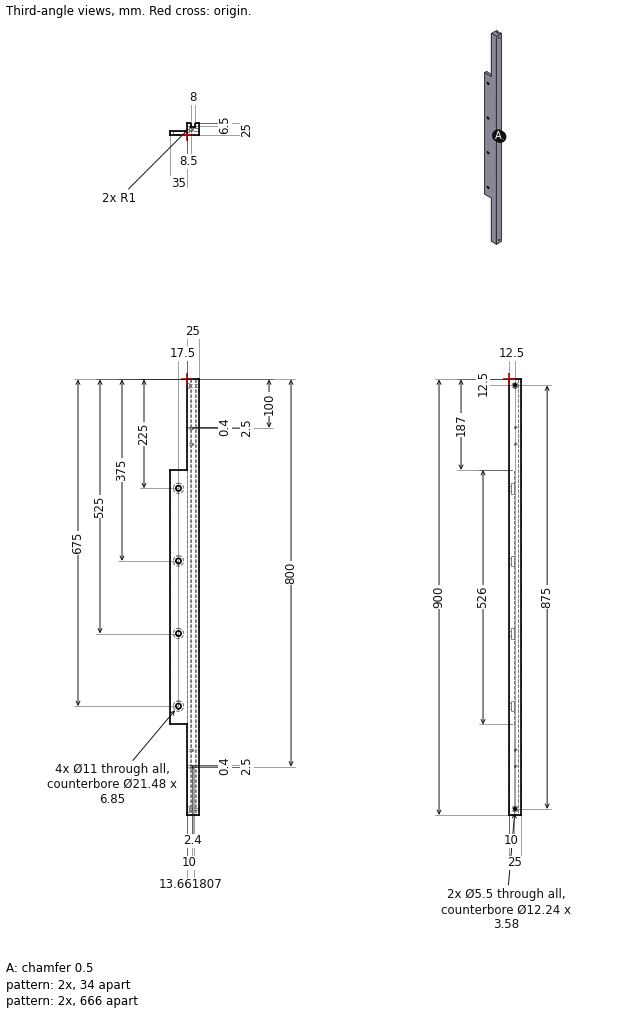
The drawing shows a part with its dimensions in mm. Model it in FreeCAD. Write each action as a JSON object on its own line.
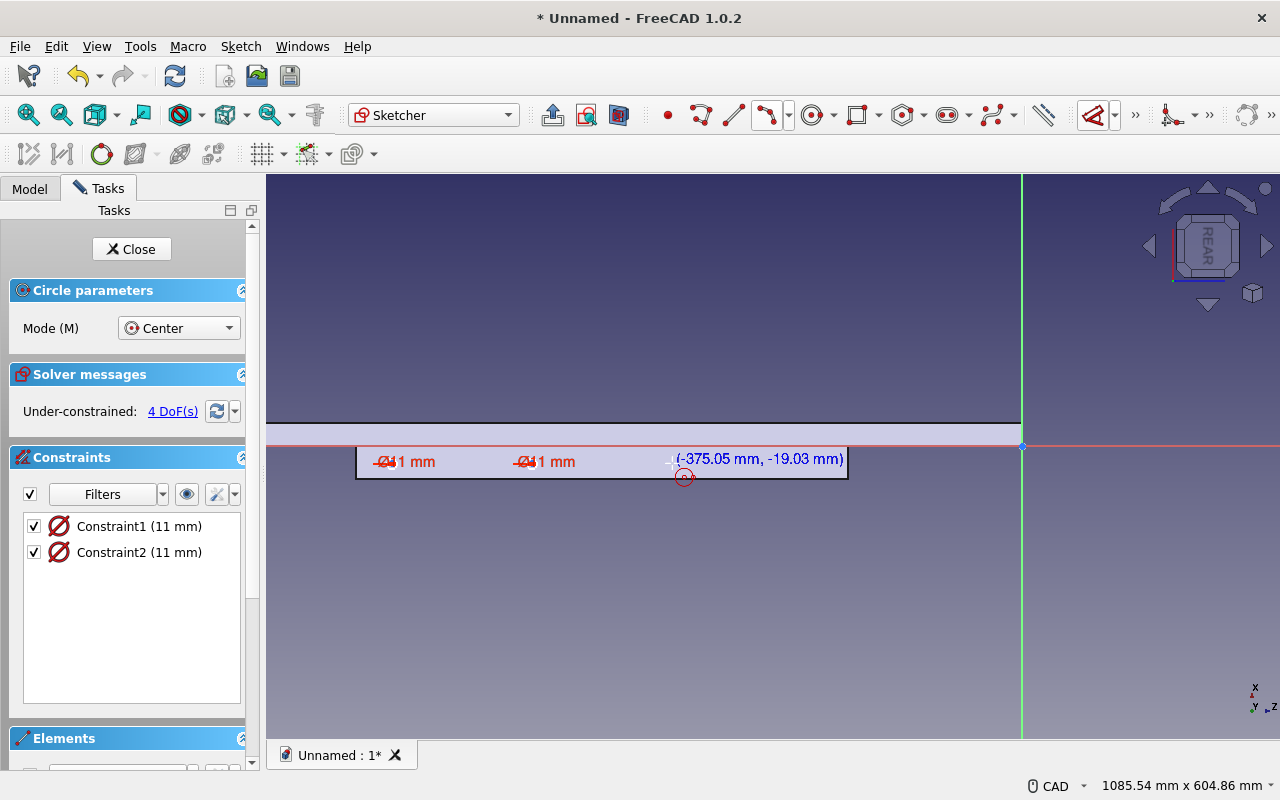
{"action": "left_click", "coordinate": [672, 463]}
{"action": "mouse_move", "coordinate": [676, 466]}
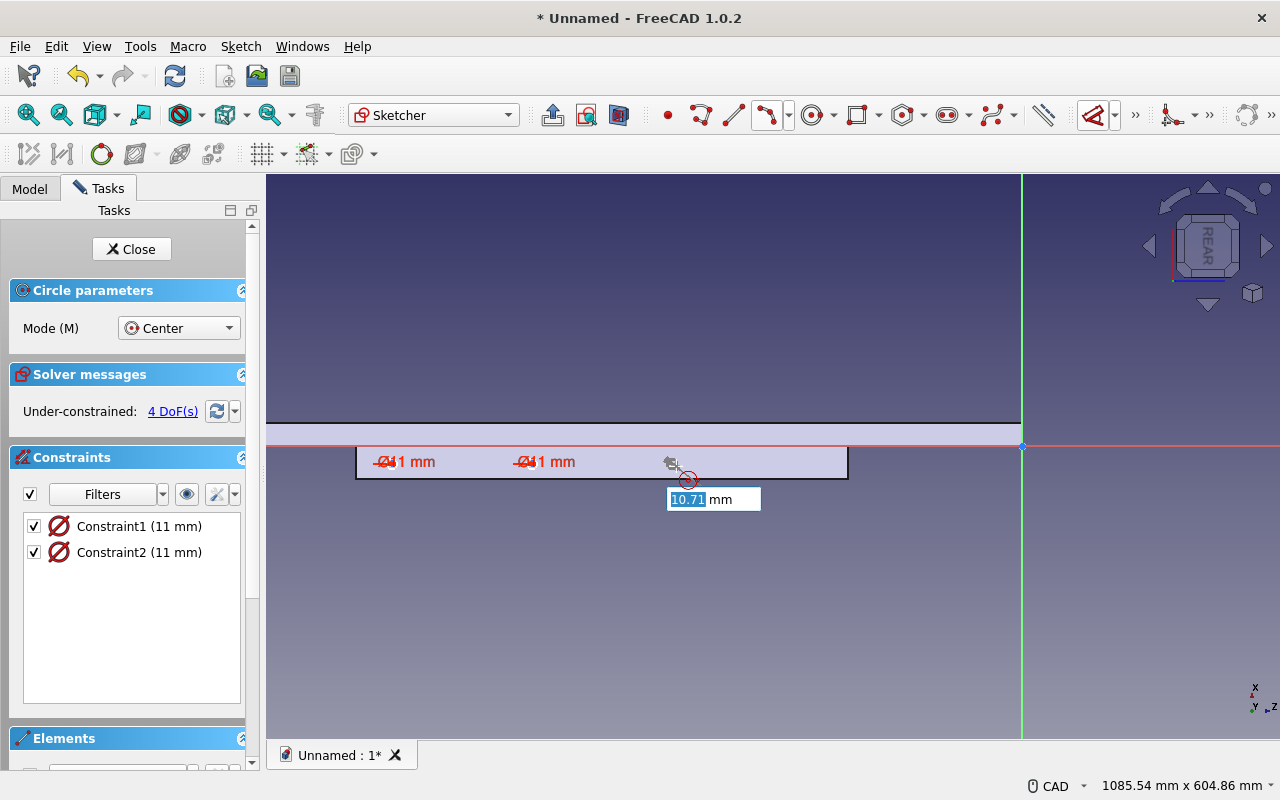
{"action": "type", "text": "11"}
{"action": "key", "text": "Return"}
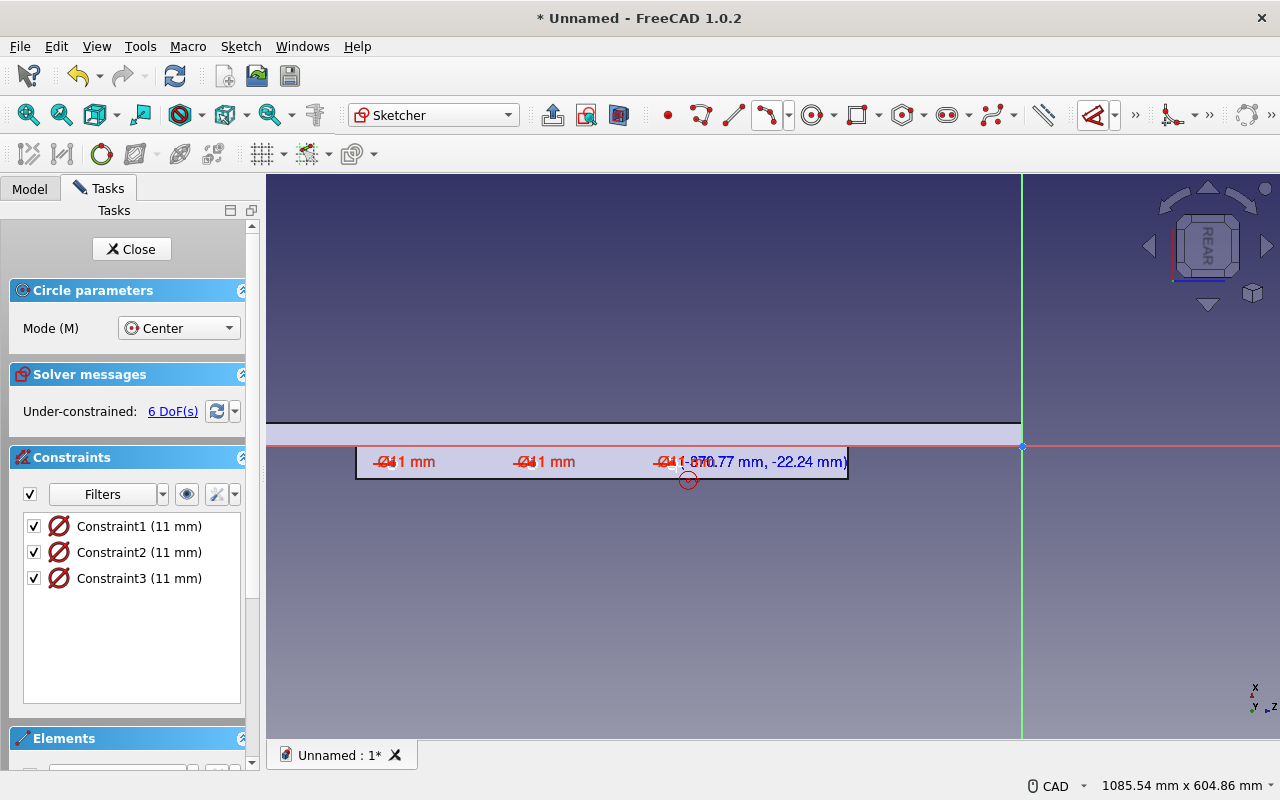
{"action": "scroll", "coordinate": [812, 463], "scroll_direction": "up", "scroll_amount": 8}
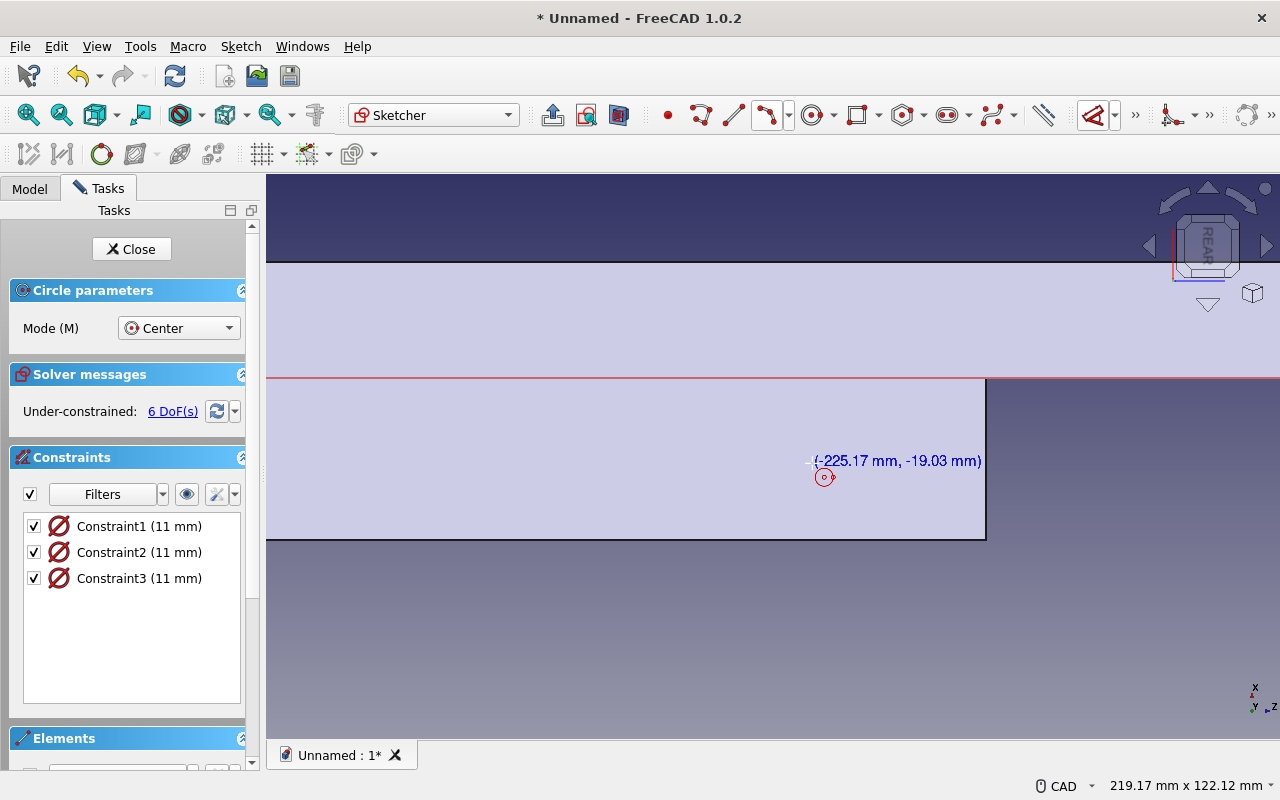
{"action": "scroll", "coordinate": [813, 463], "scroll_direction": "down", "scroll_amount": 8}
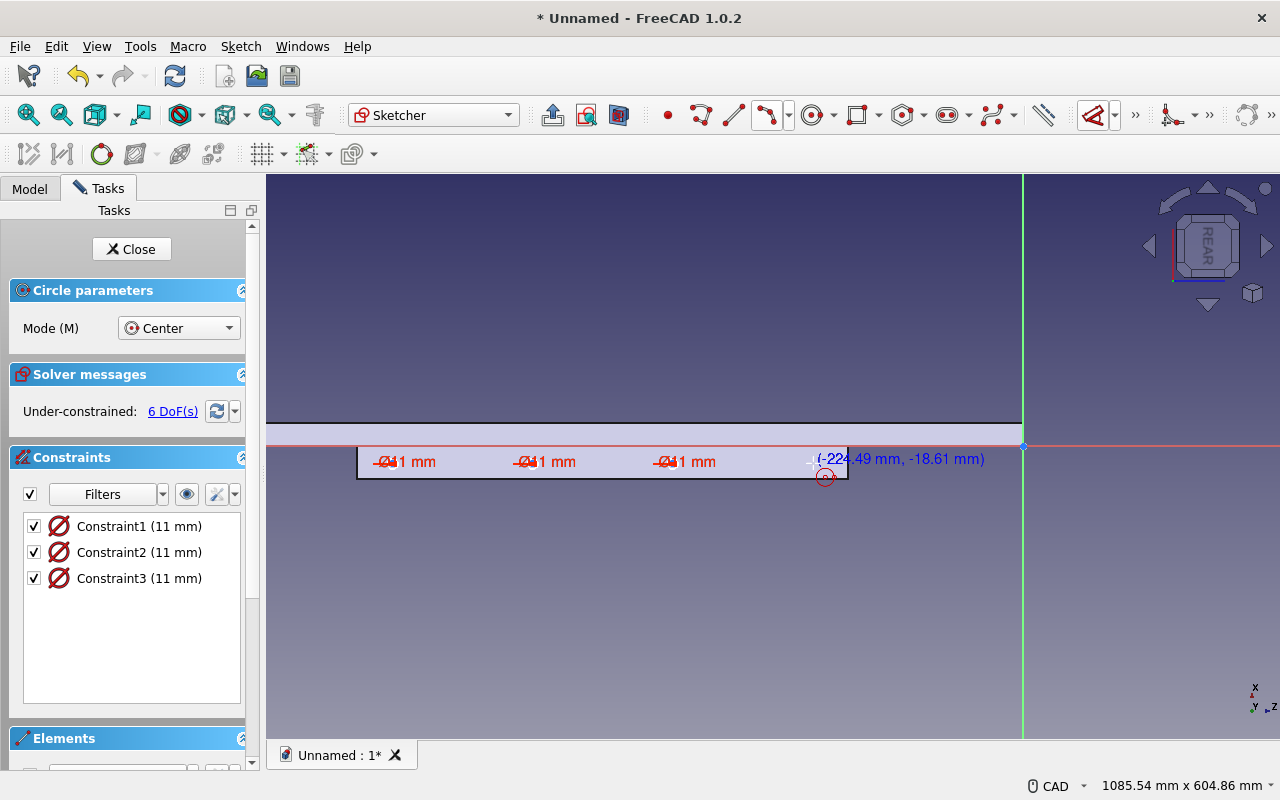
{"action": "left_click", "coordinate": [813, 463]}
{"action": "mouse_move", "coordinate": [817, 466]}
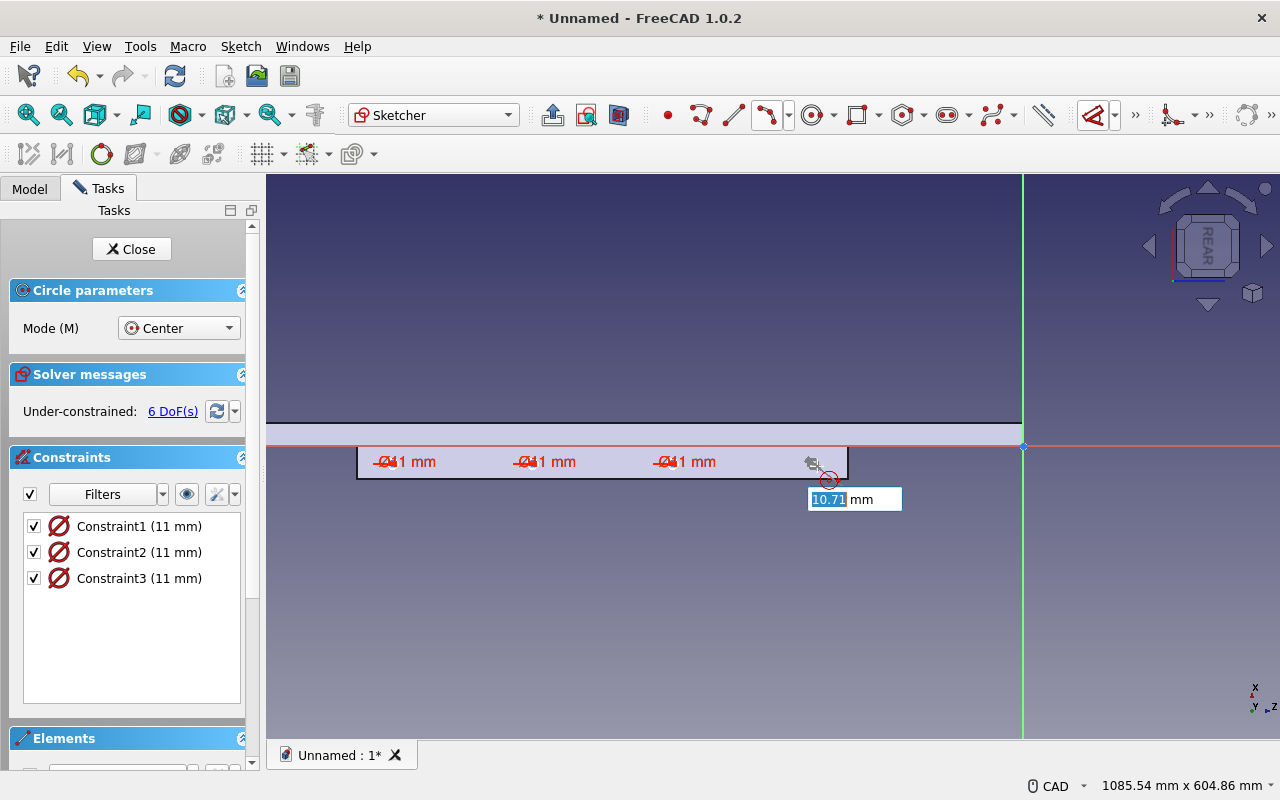
{"action": "type", "text": "11"}
{"action": "key", "text": "Return"}
{"action": "key", "text": "Escape"}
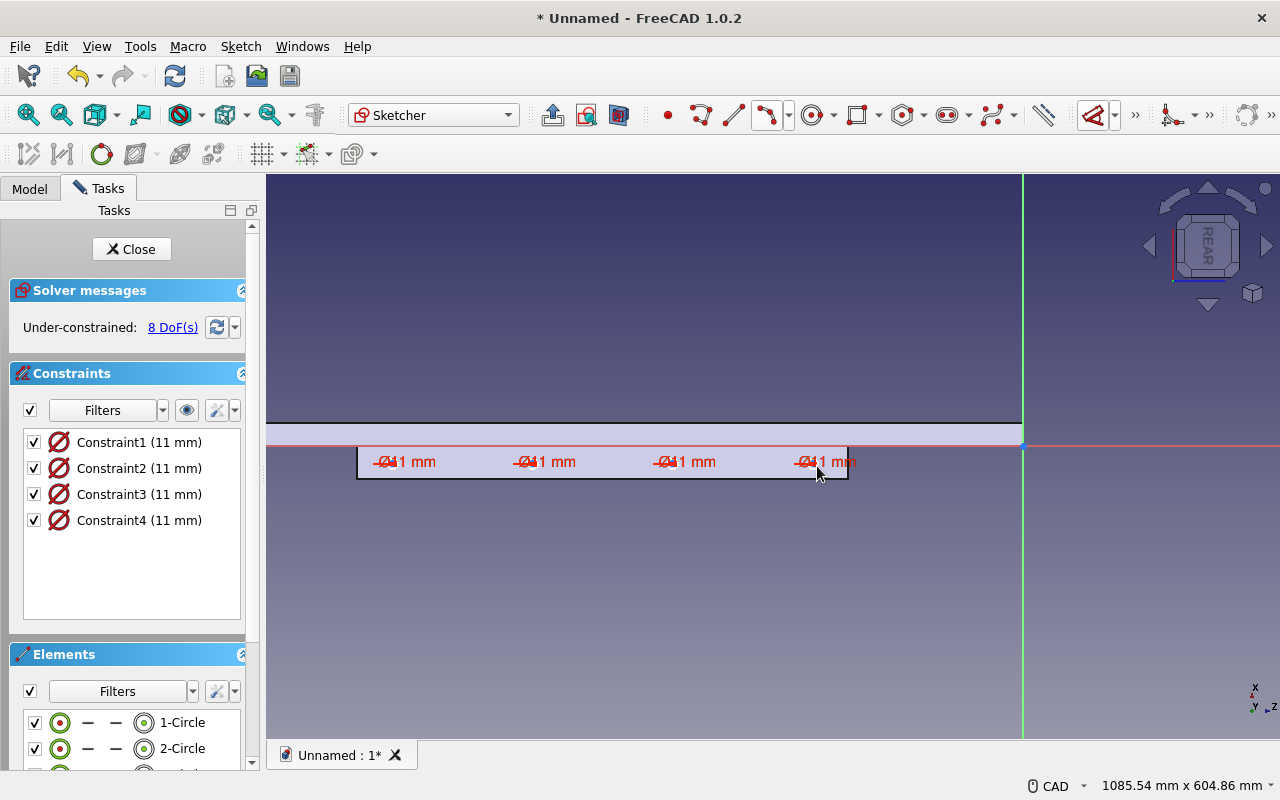
{"action": "left_click", "coordinate": [393, 464]}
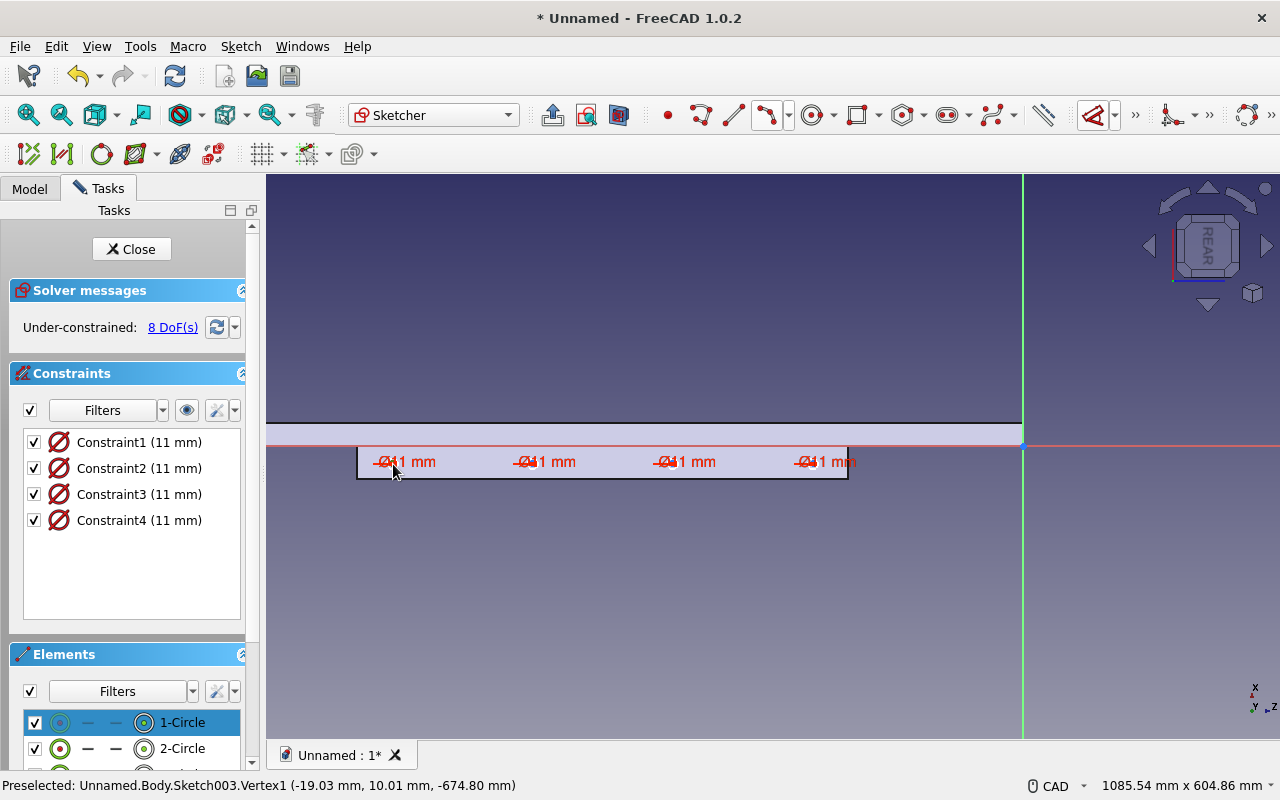
{"action": "left_click", "coordinate": [533, 464]}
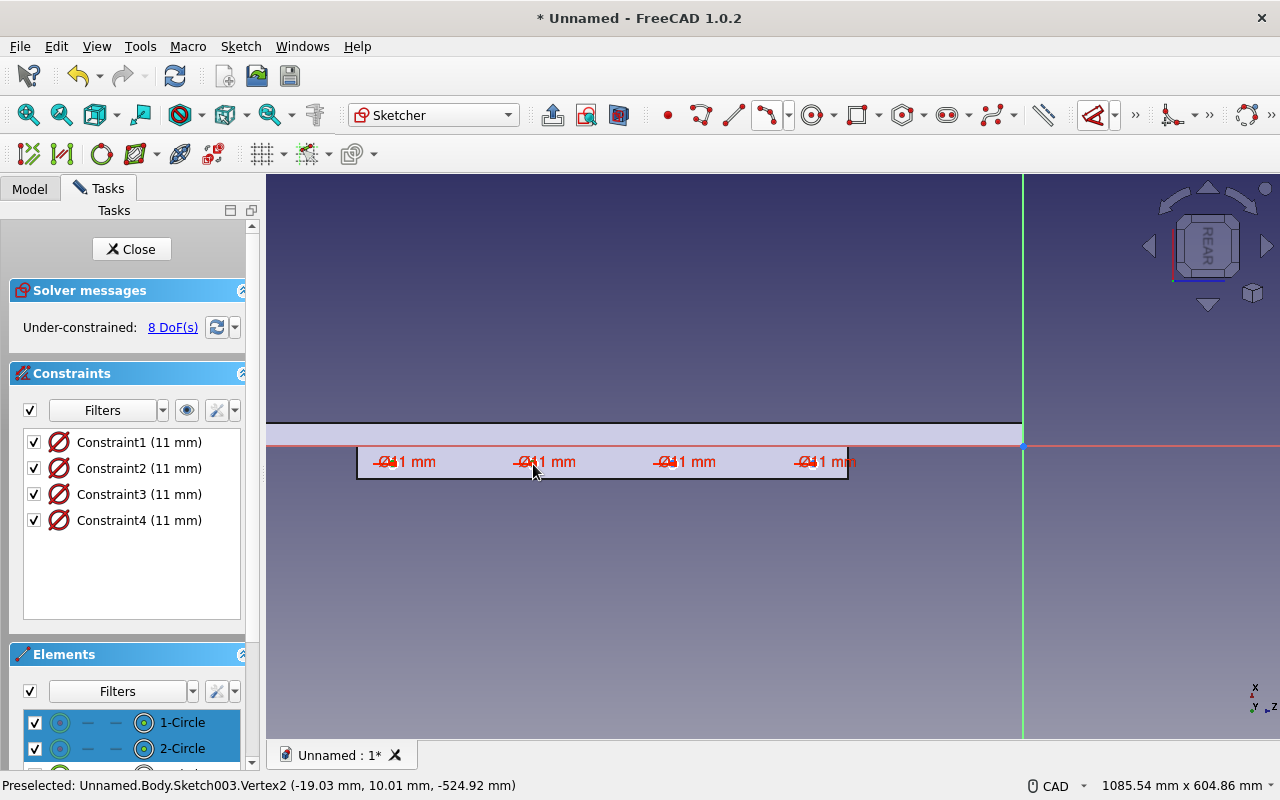
{"action": "key", "text": "h"}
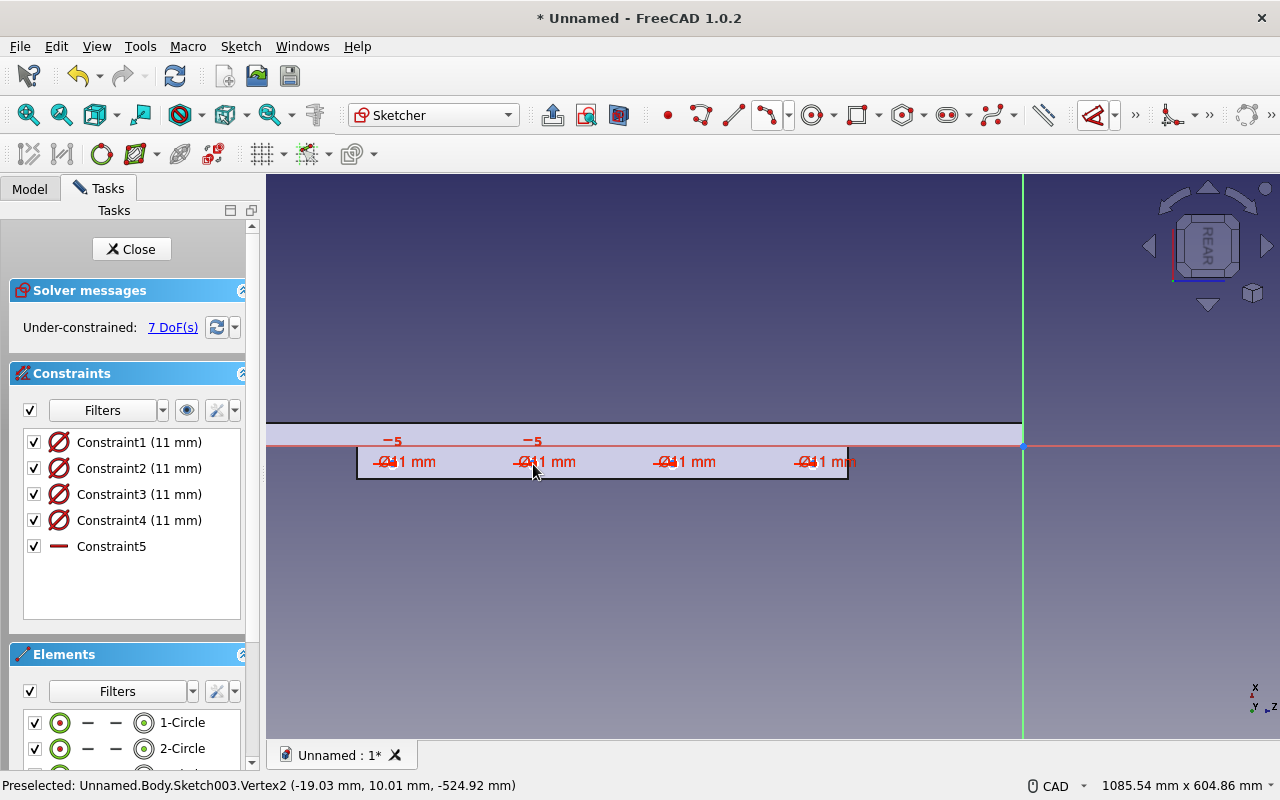
{"action": "left_click", "coordinate": [533, 464]}